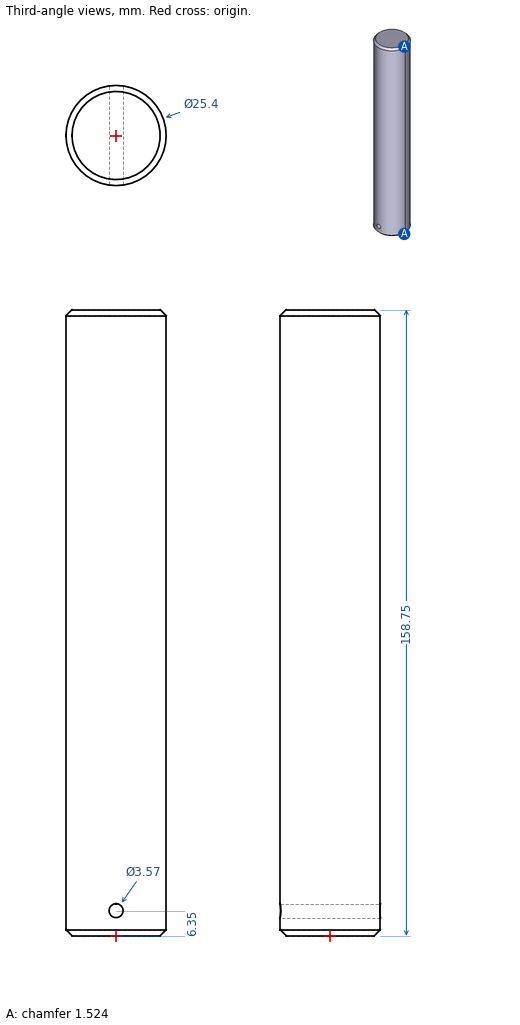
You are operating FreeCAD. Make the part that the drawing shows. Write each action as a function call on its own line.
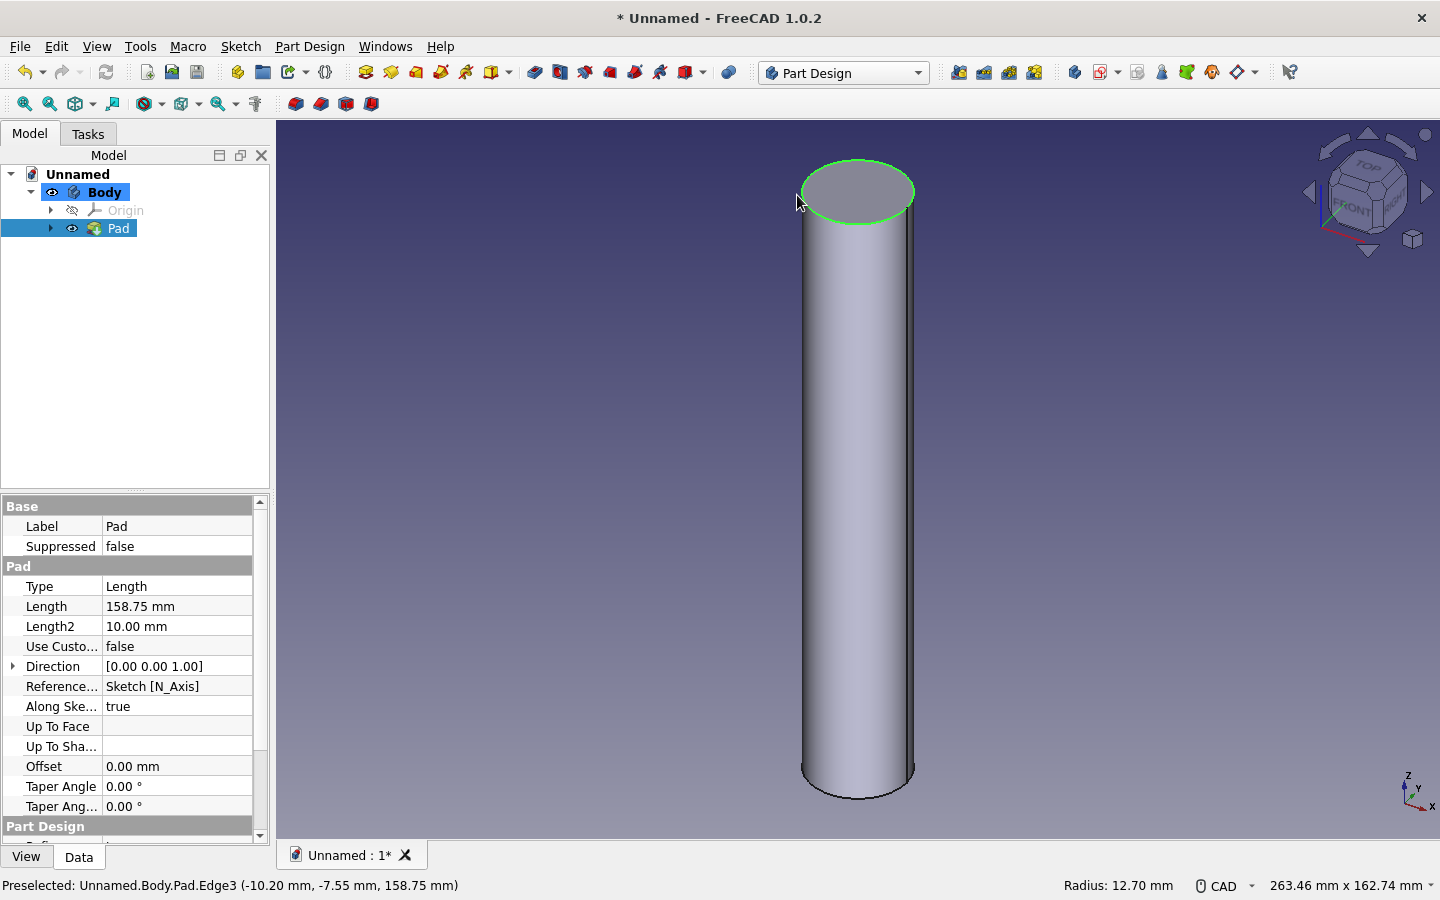
key(0)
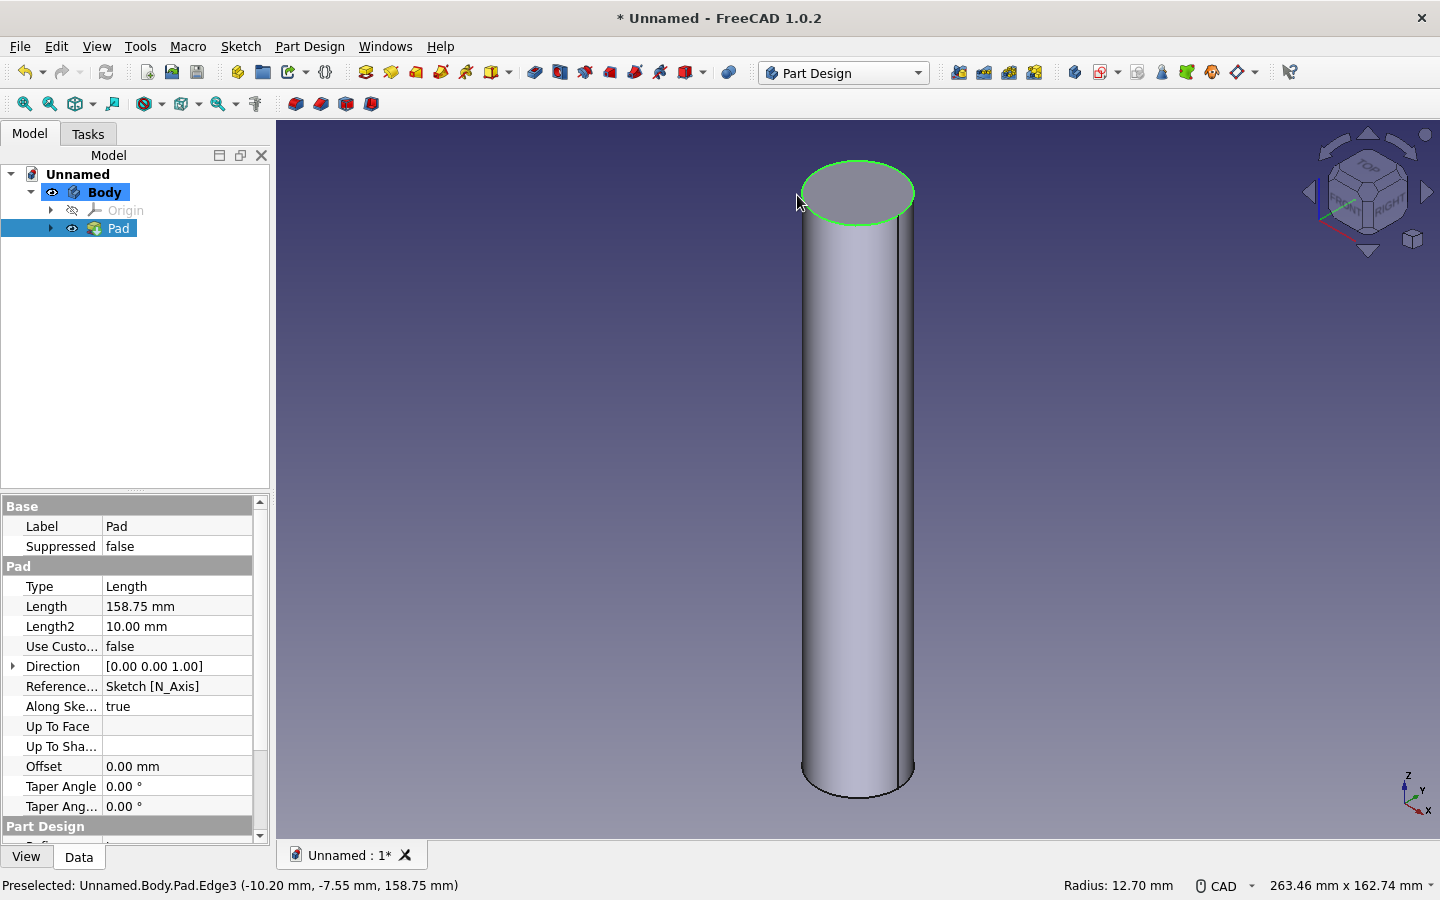
key(2)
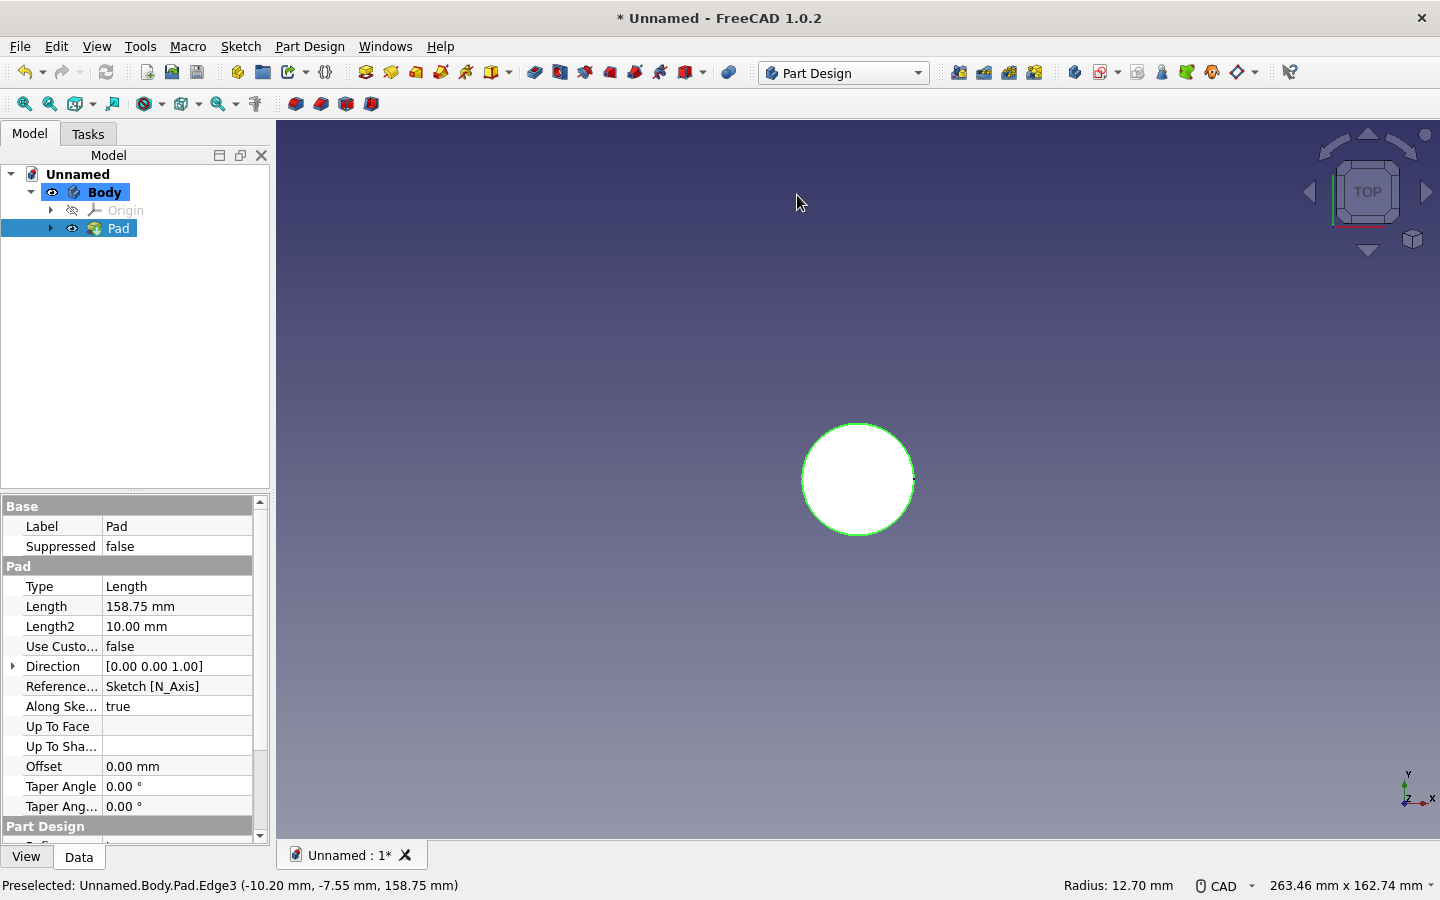
key(v)
key(f)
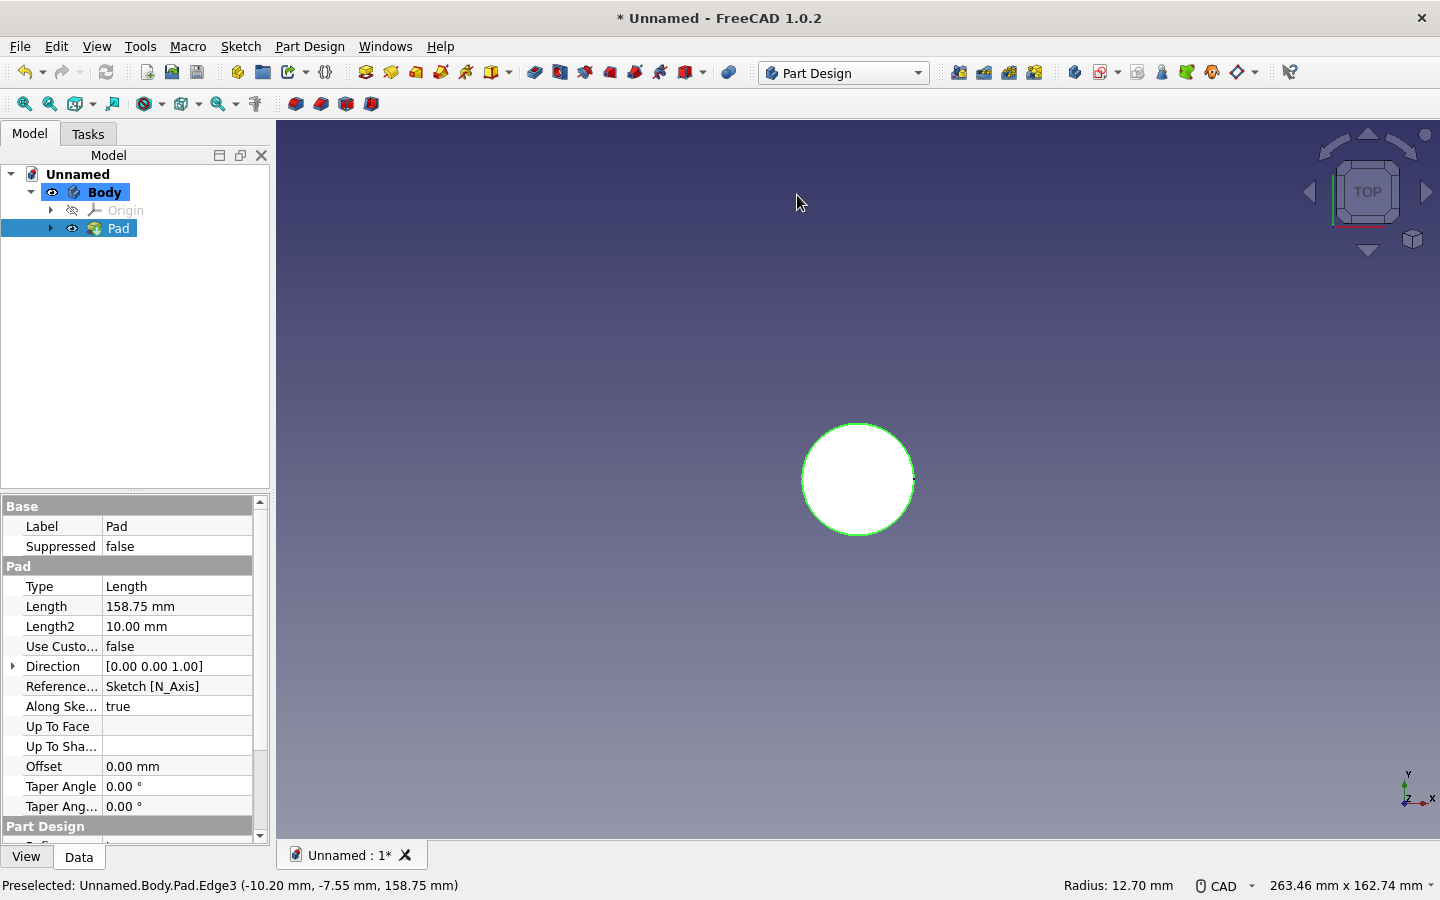
key(1)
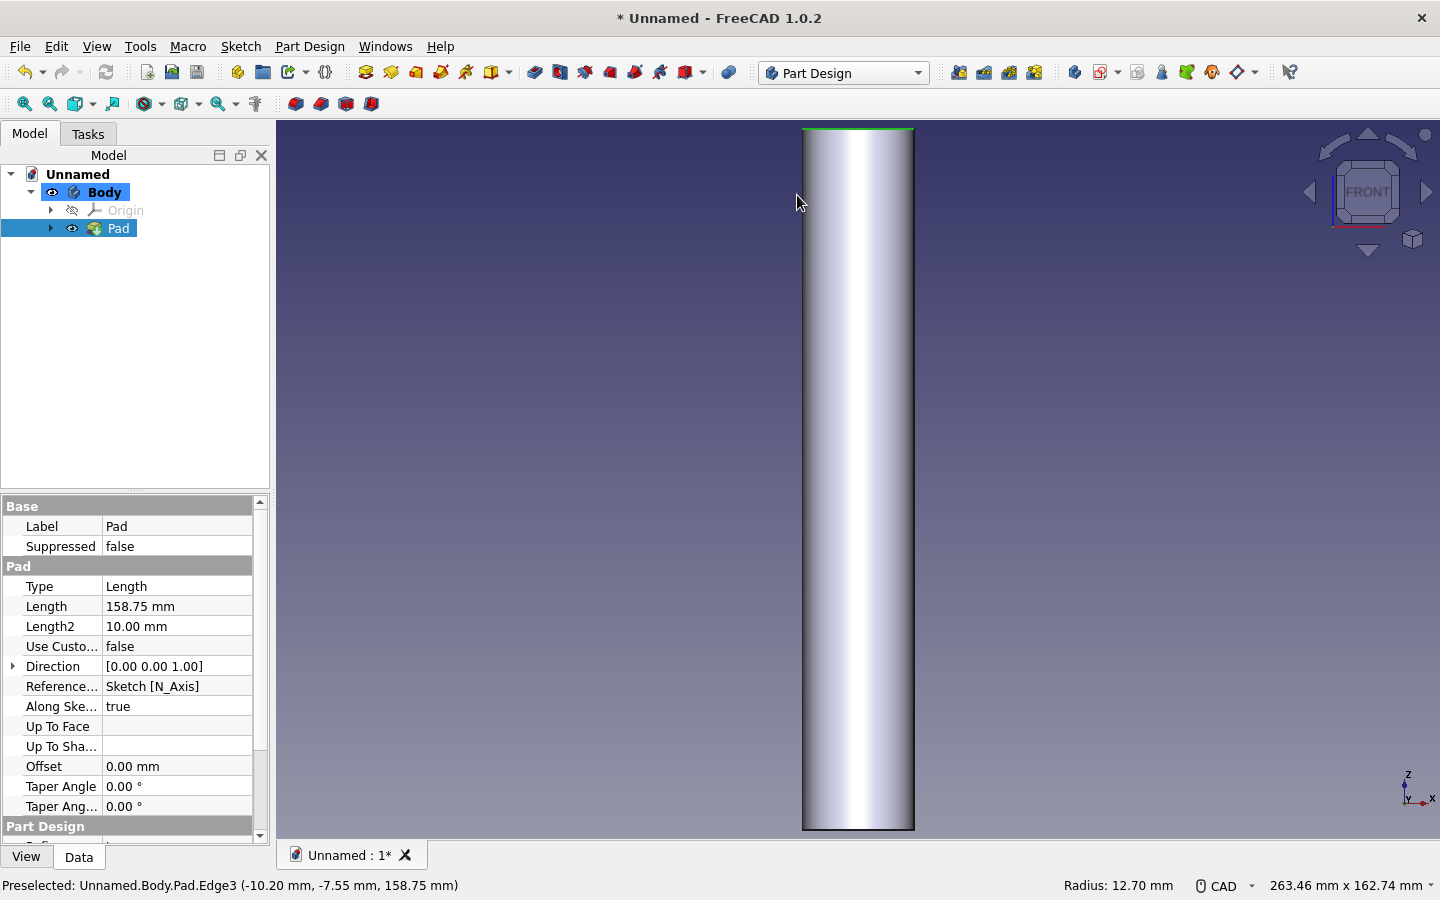
key(3)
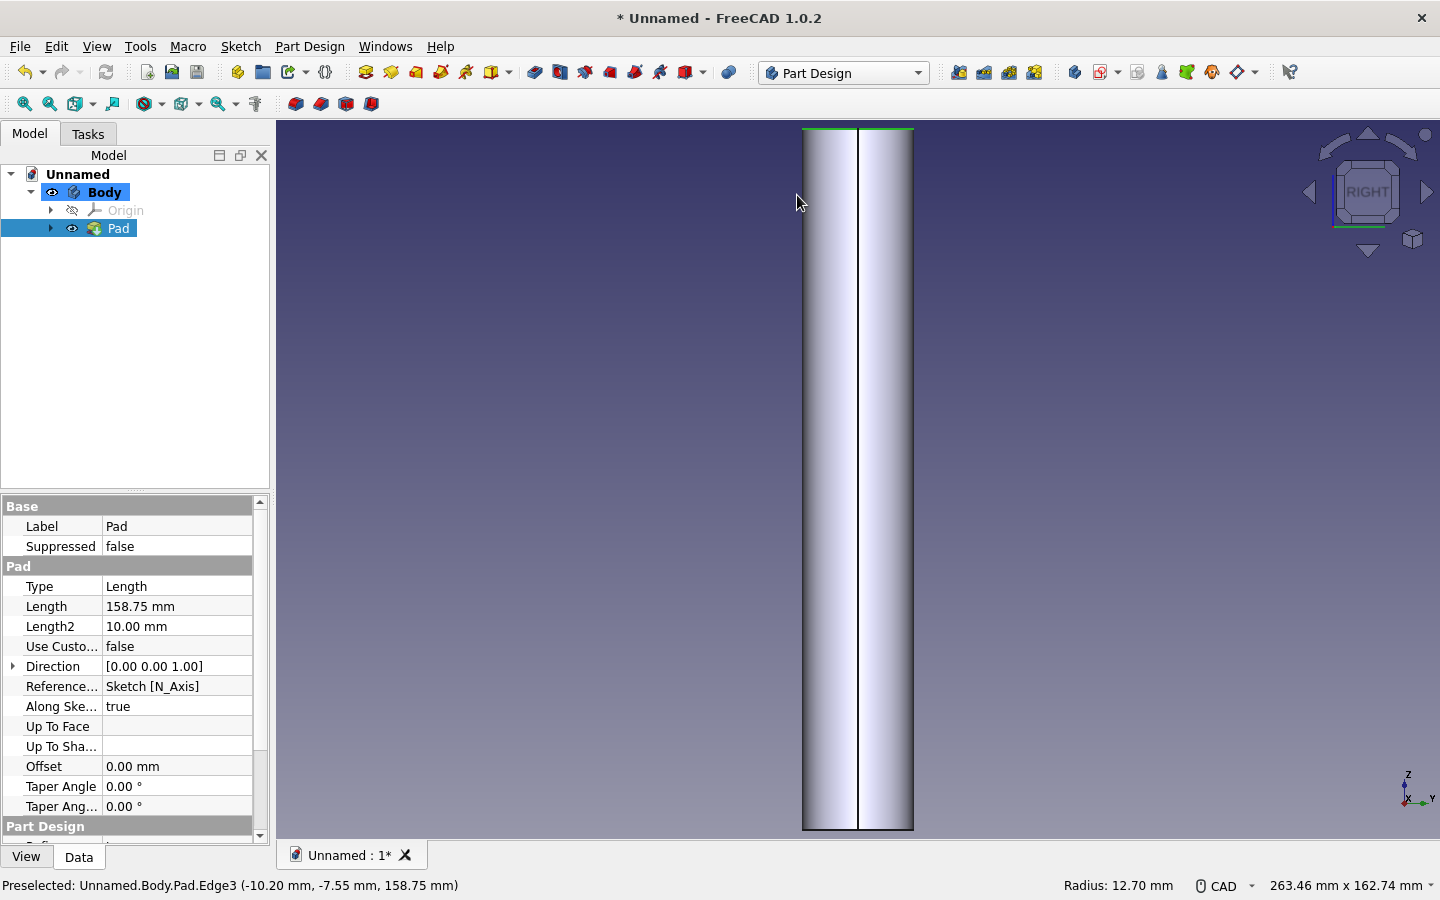
key(5)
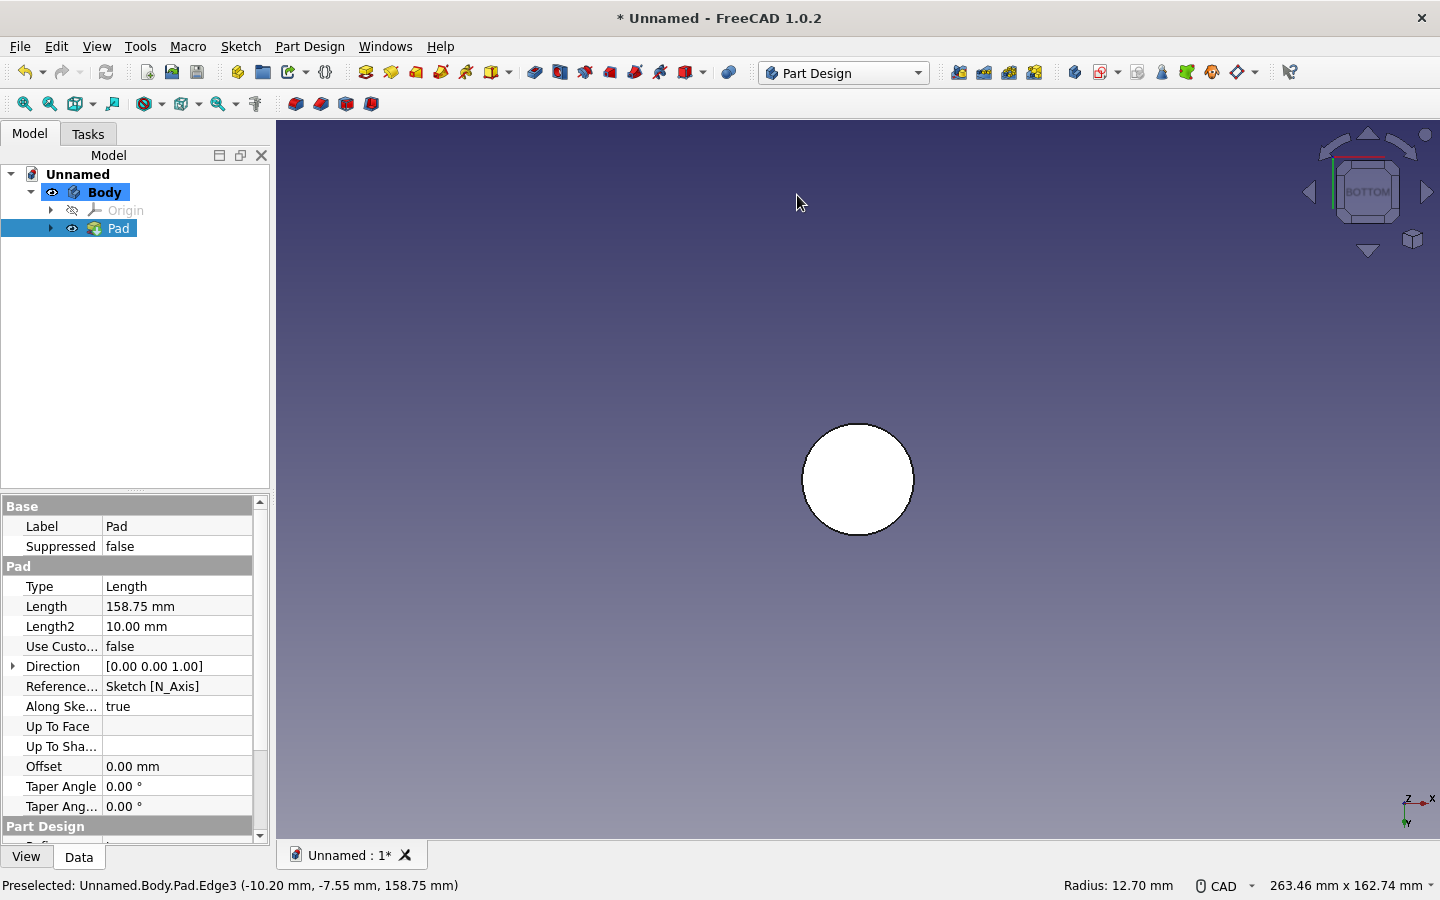
key(v)
key(f)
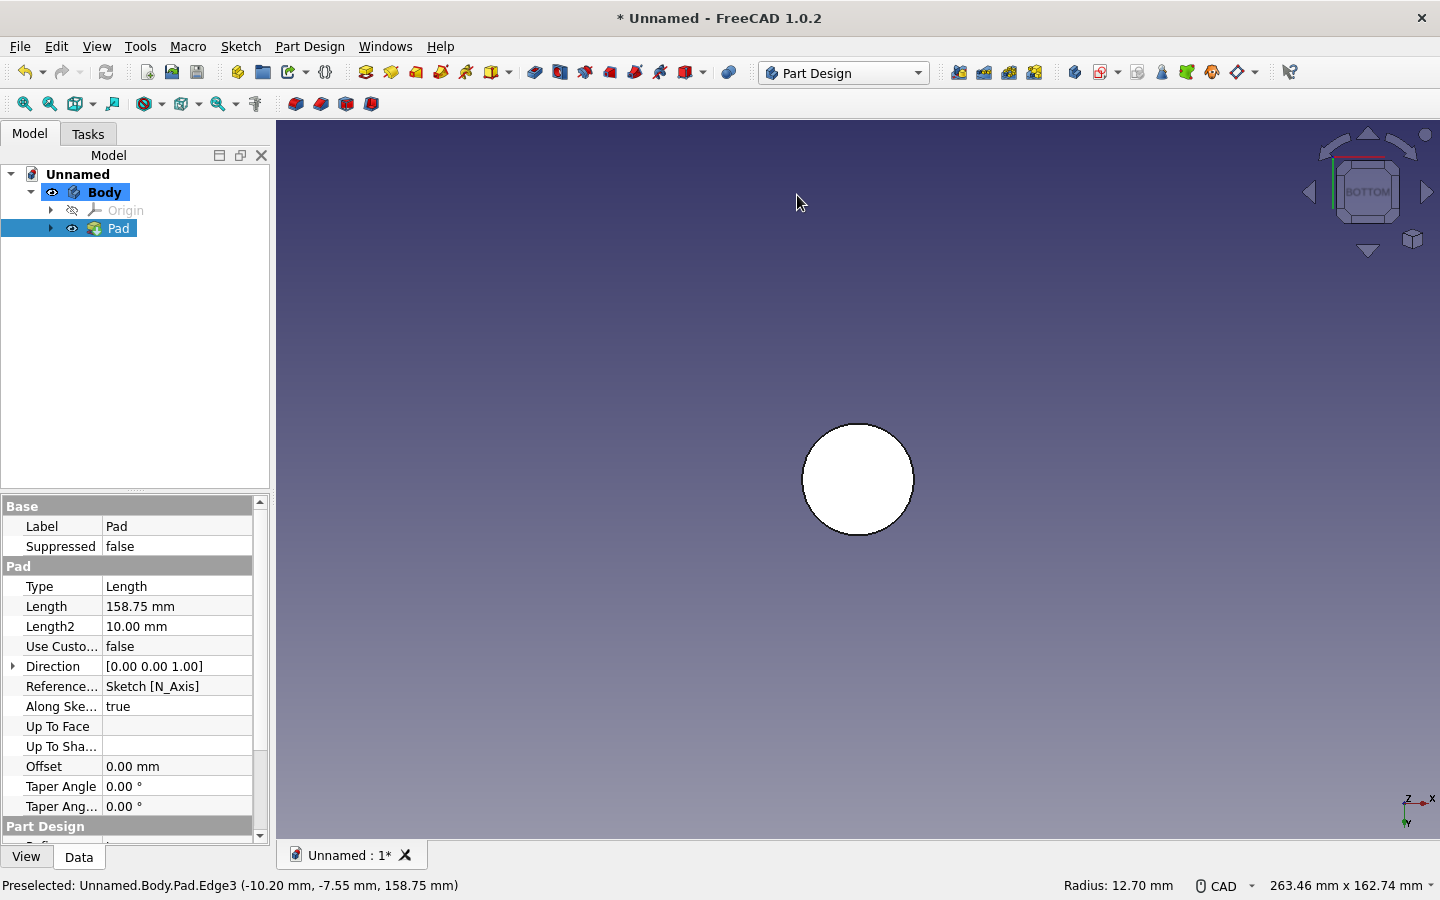
click(802, 478, ctrl)